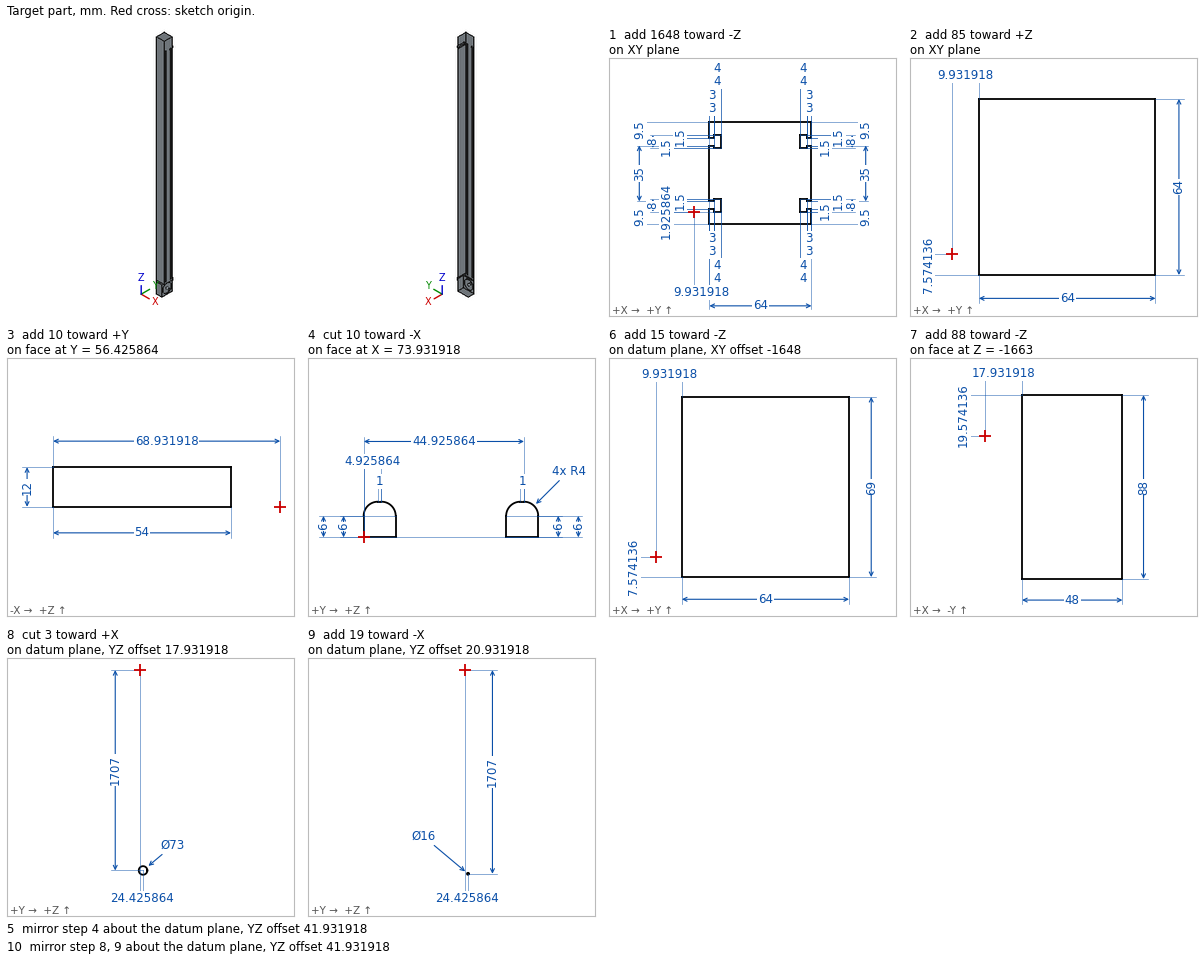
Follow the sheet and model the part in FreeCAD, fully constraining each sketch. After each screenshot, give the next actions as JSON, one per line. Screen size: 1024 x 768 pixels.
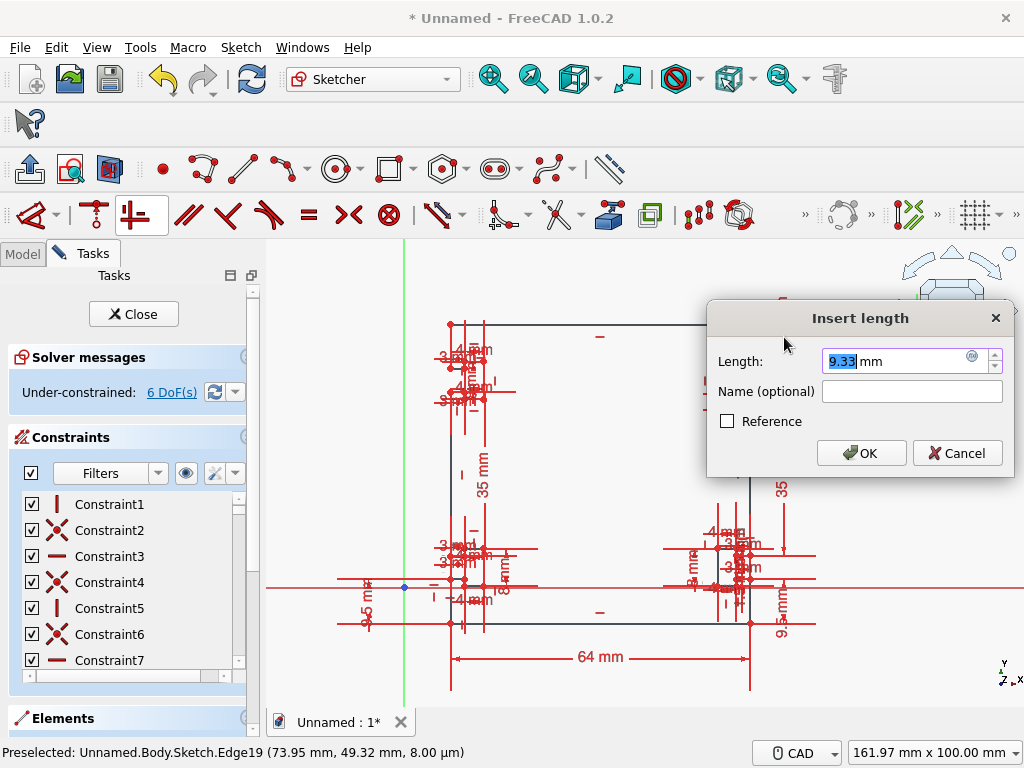
{"action": "type", "text": "9.5"}
{"action": "key", "text": "Return"}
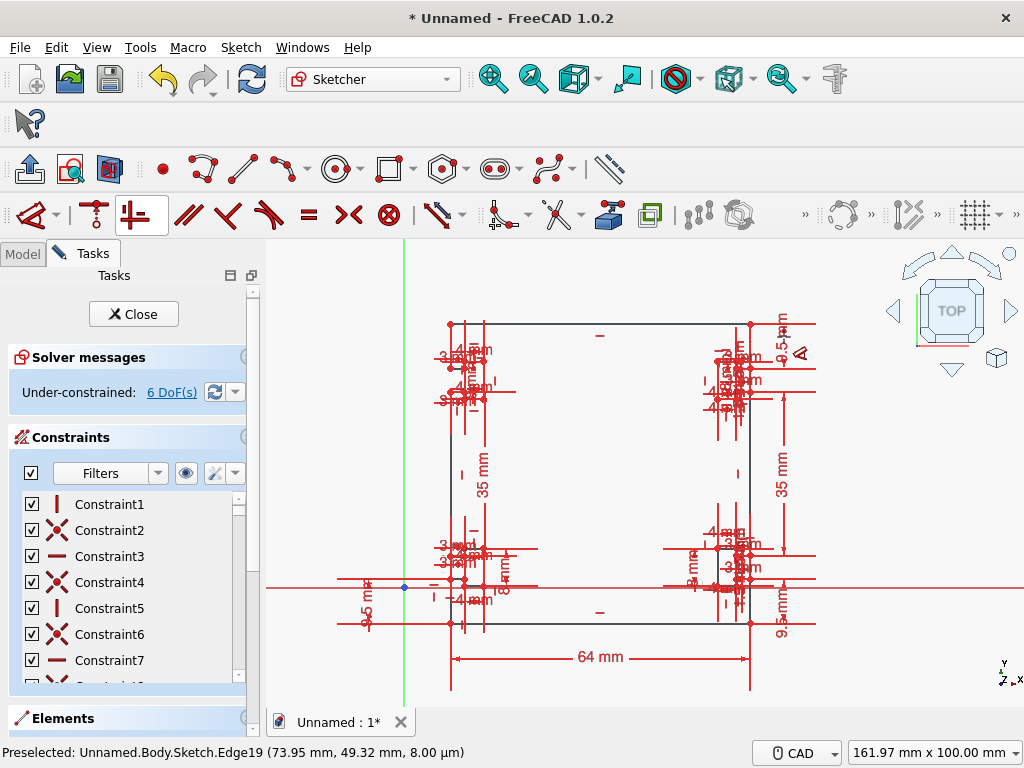
{"action": "left_click", "coordinate": [451, 338]}
{"action": "left_click", "coordinate": [369, 347]}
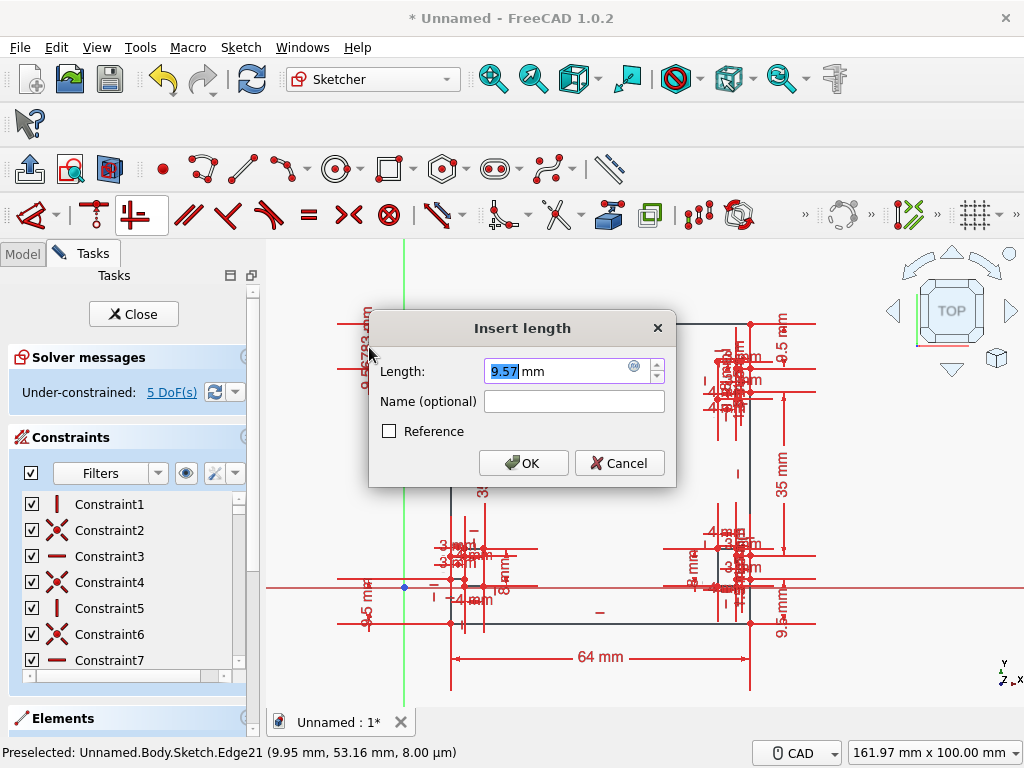
{"action": "type", "text": "9.5"}
{"action": "key", "text": "Return"}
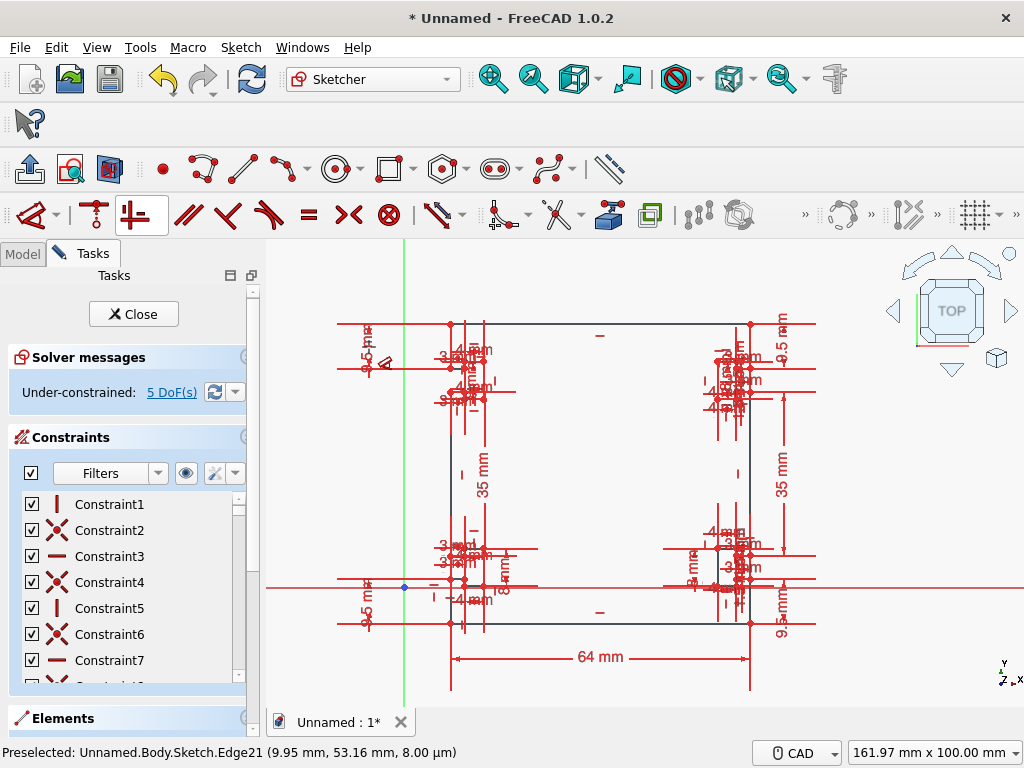
{"action": "scroll", "coordinate": [465, 365], "scroll_direction": "up", "scroll_amount": 9}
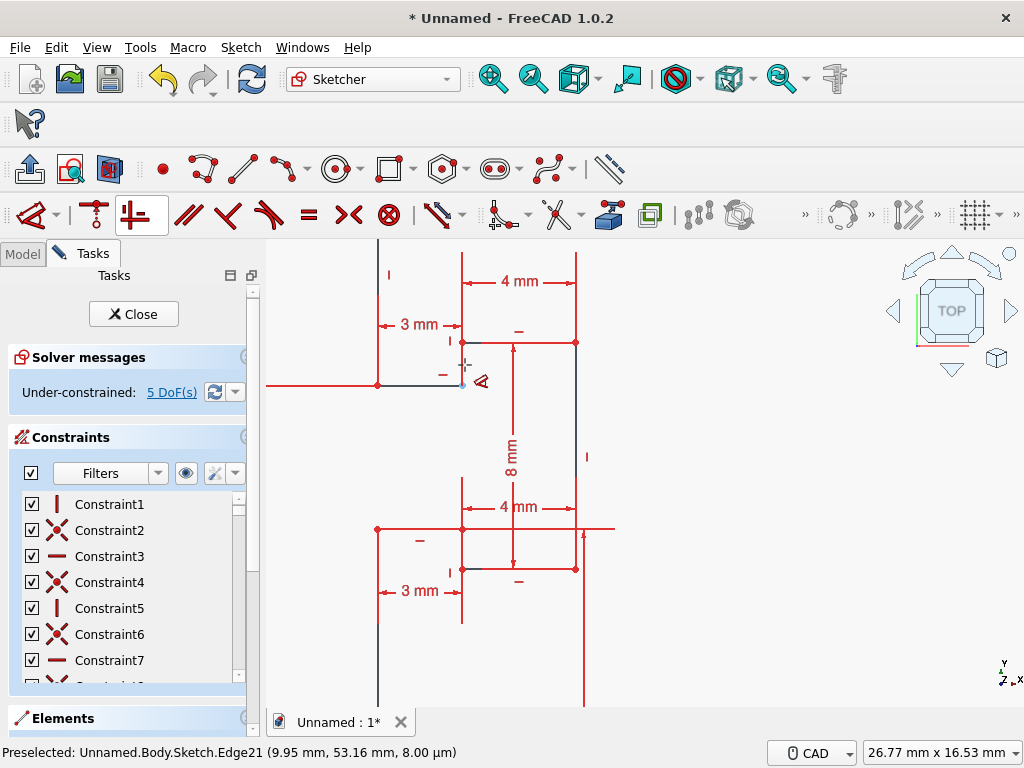
{"action": "left_click", "coordinate": [462, 364]}
{"action": "left_click", "coordinate": [428, 364]}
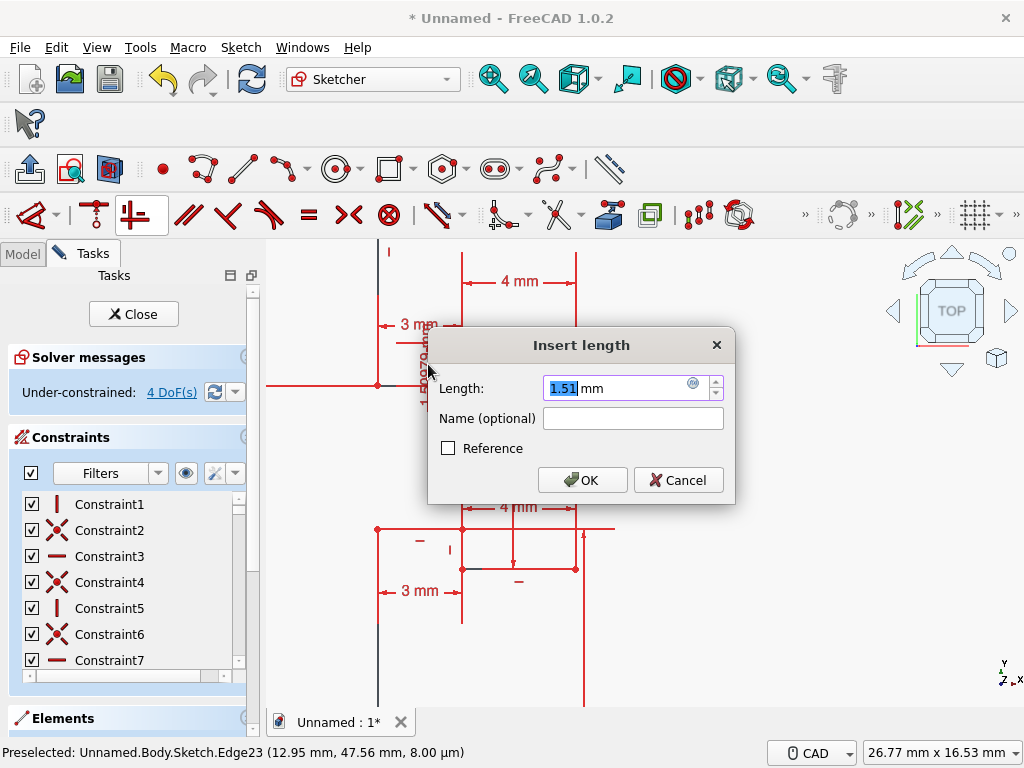
{"action": "type", "text": "1.5"}
{"action": "key", "text": "Return"}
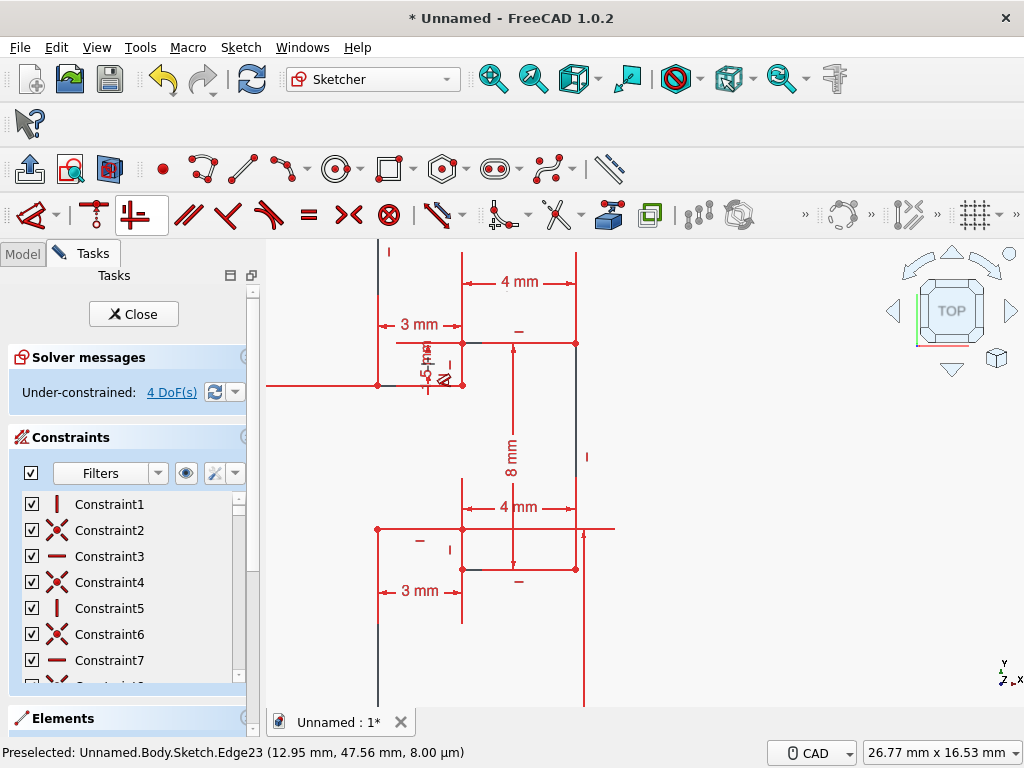
{"action": "left_click", "coordinate": [462, 558]}
{"action": "left_click", "coordinate": [428, 549]}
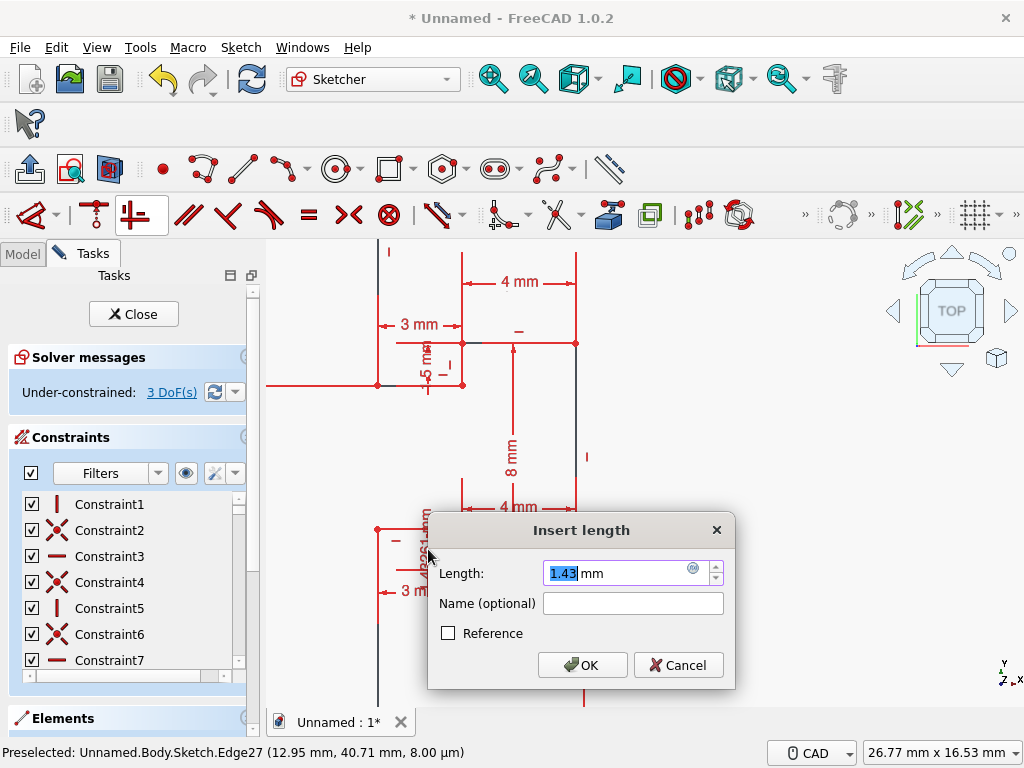
{"action": "type", "text": "1.5"}
{"action": "key", "text": "Return"}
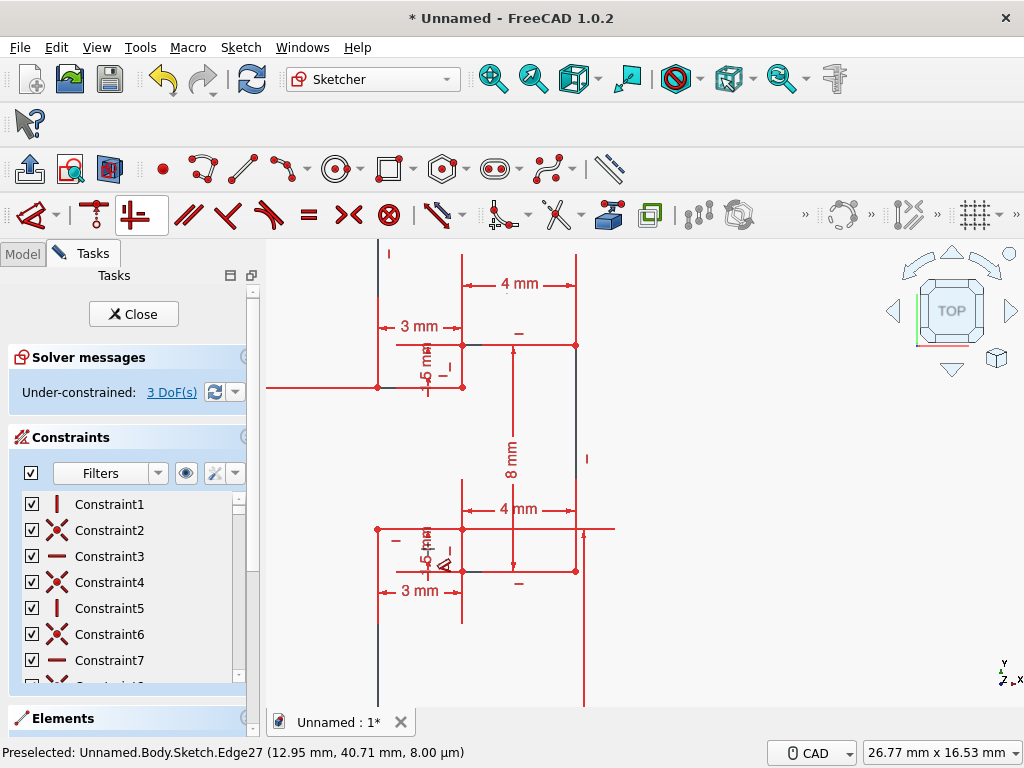
{"action": "scroll", "coordinate": [464, 365], "scroll_direction": "down", "scroll_amount": 9}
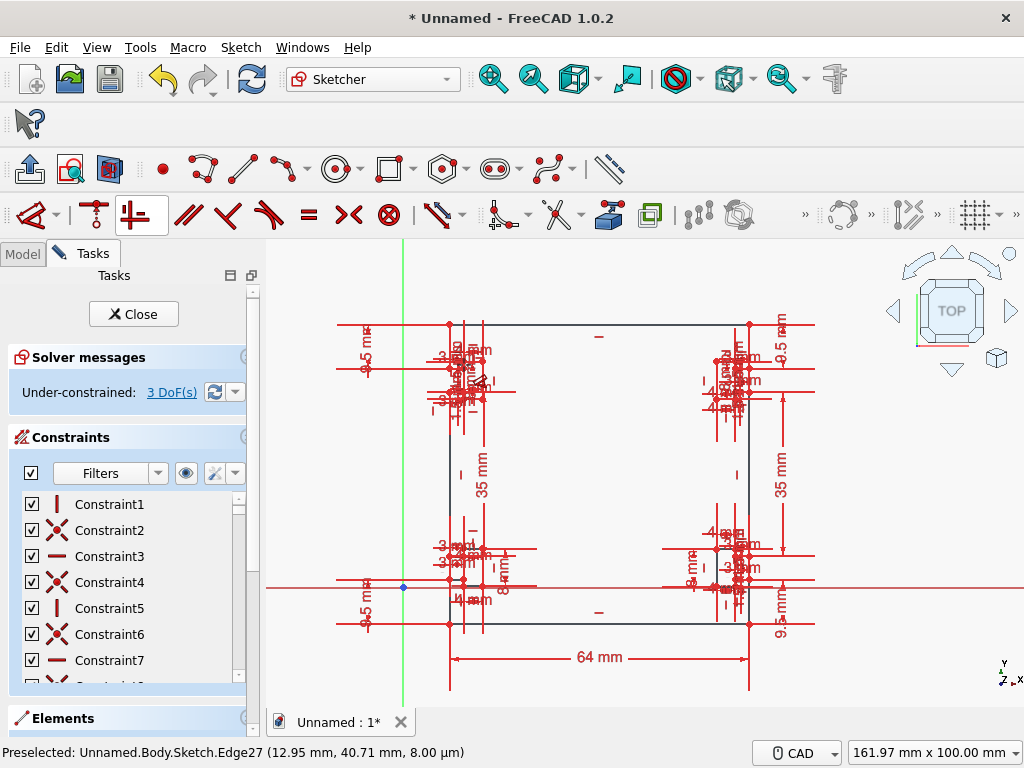
{"action": "scroll", "coordinate": [464, 554], "scroll_direction": "up", "scroll_amount": 10}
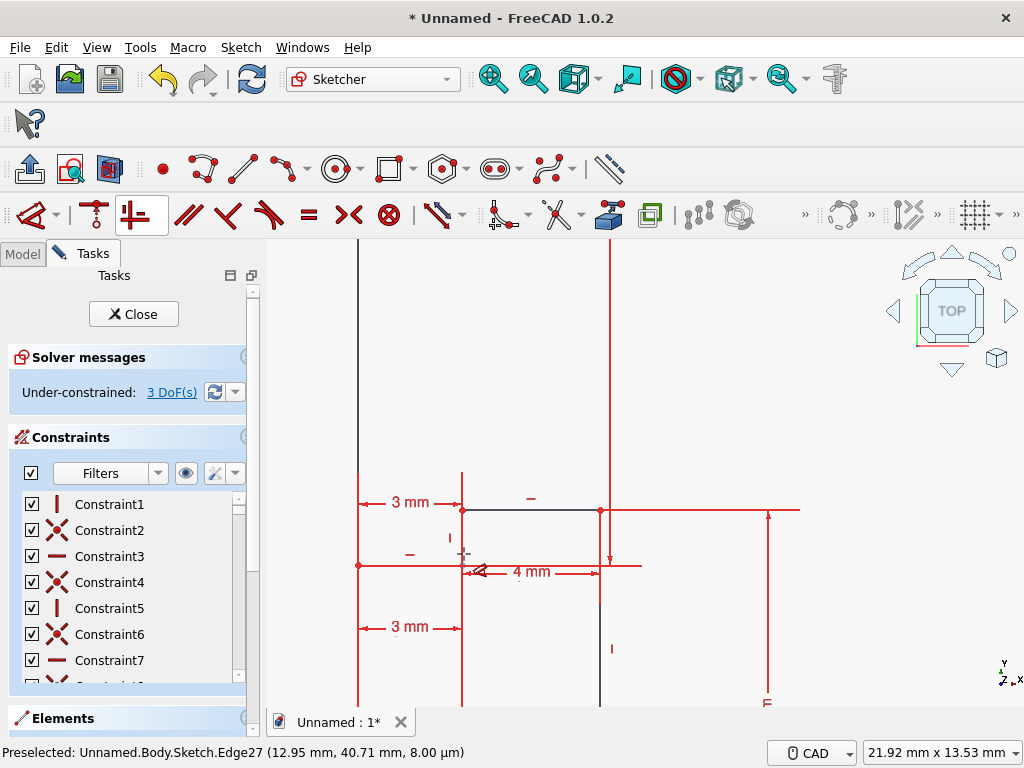
{"action": "left_click", "coordinate": [462, 549]}
{"action": "left_click", "coordinate": [428, 538]}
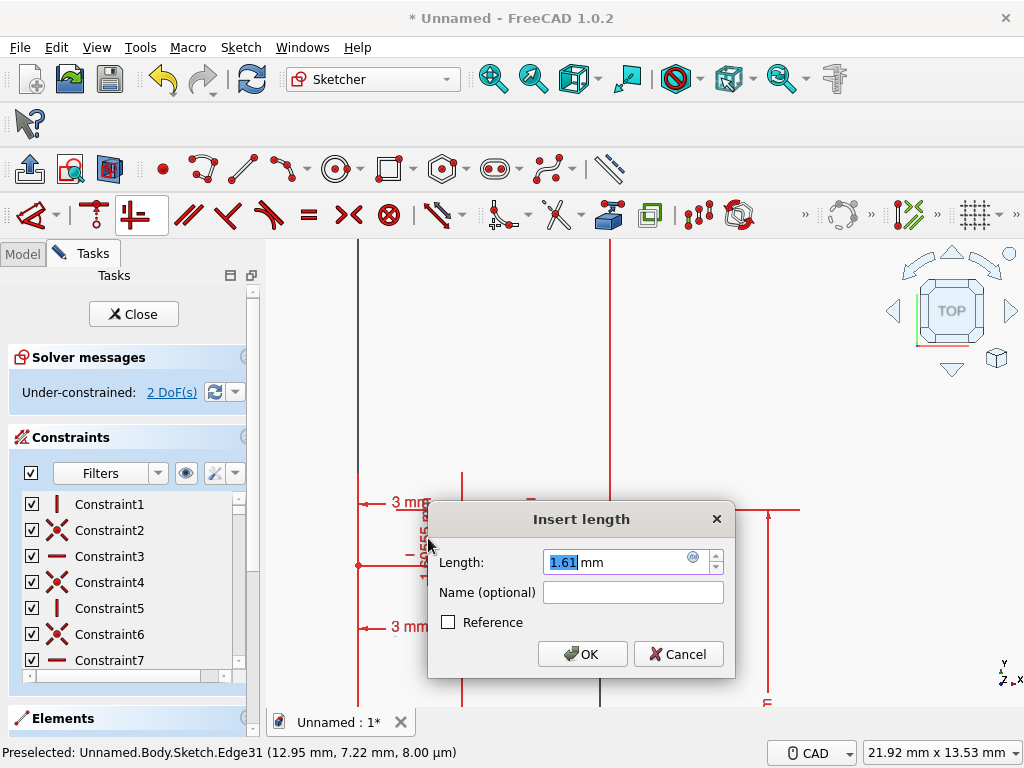
{"action": "type", "text": "1.5"}
{"action": "key", "text": "Return"}